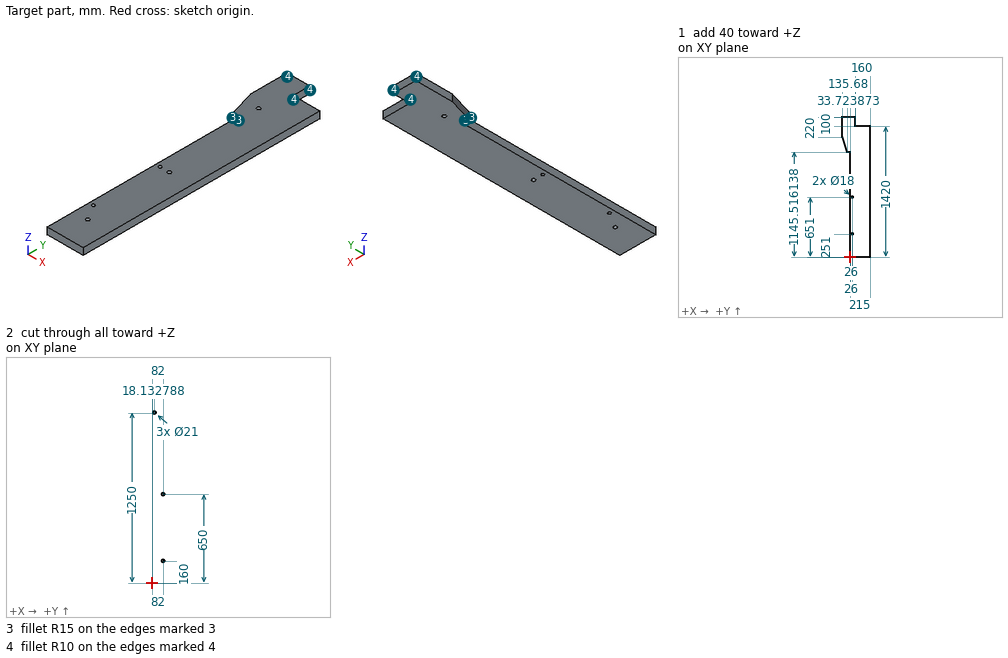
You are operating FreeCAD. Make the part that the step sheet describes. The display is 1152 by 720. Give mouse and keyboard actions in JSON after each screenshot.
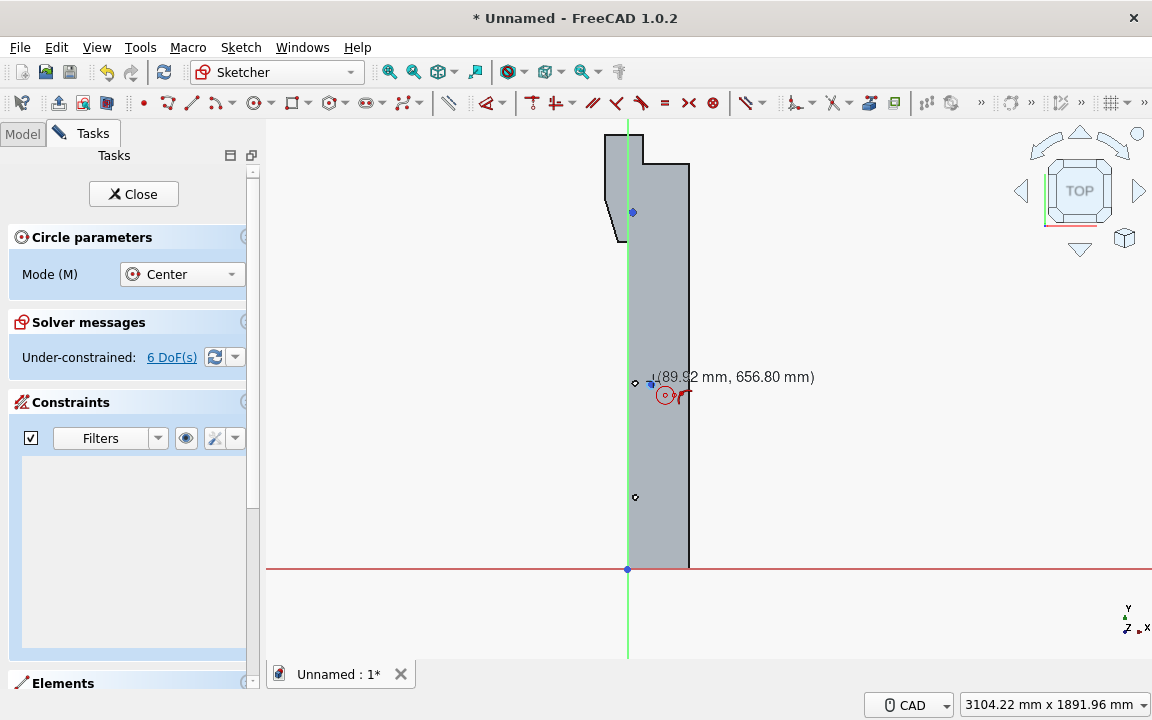
{"action": "scroll", "coordinate": [651, 523], "scroll_direction": "up", "scroll_amount": 11}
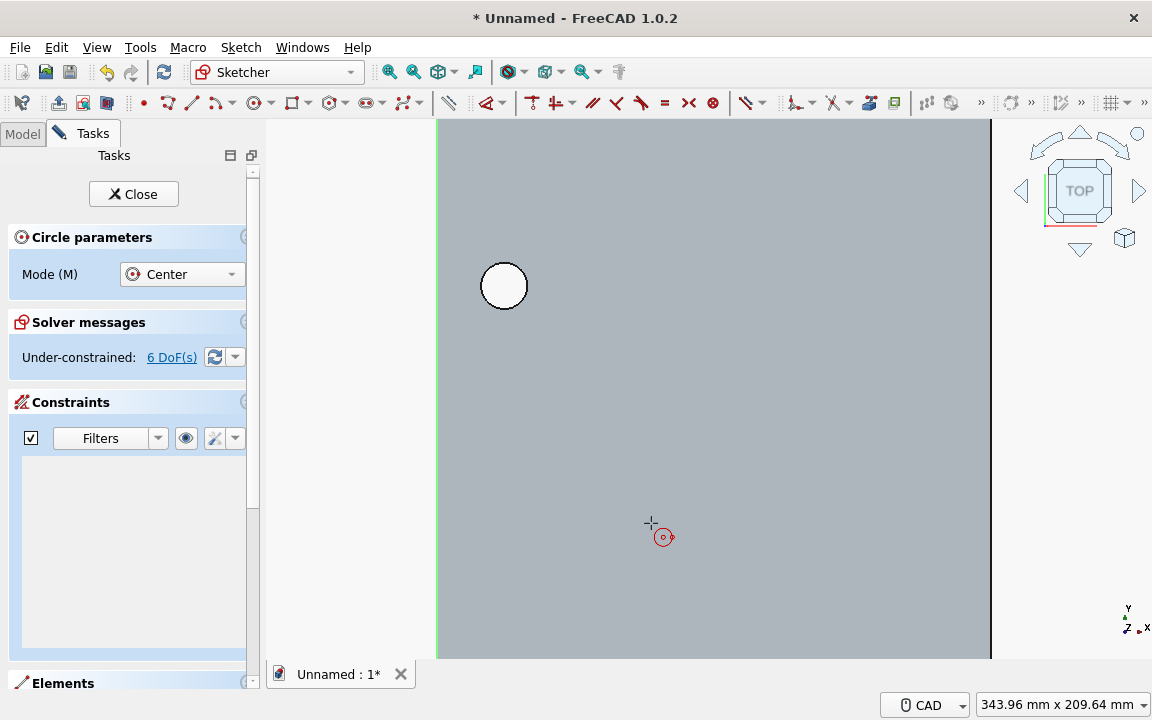
{"action": "scroll", "coordinate": [651, 524], "scroll_direction": "down", "scroll_amount": 11}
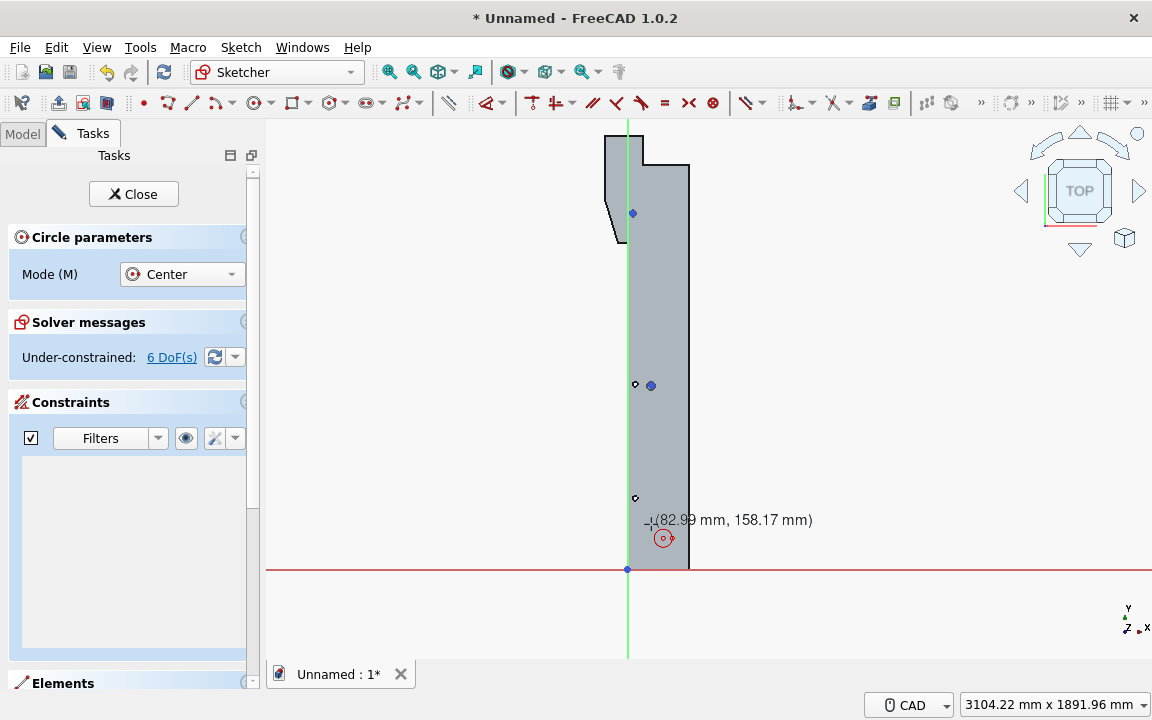
{"action": "left_click", "coordinate": [651, 524]}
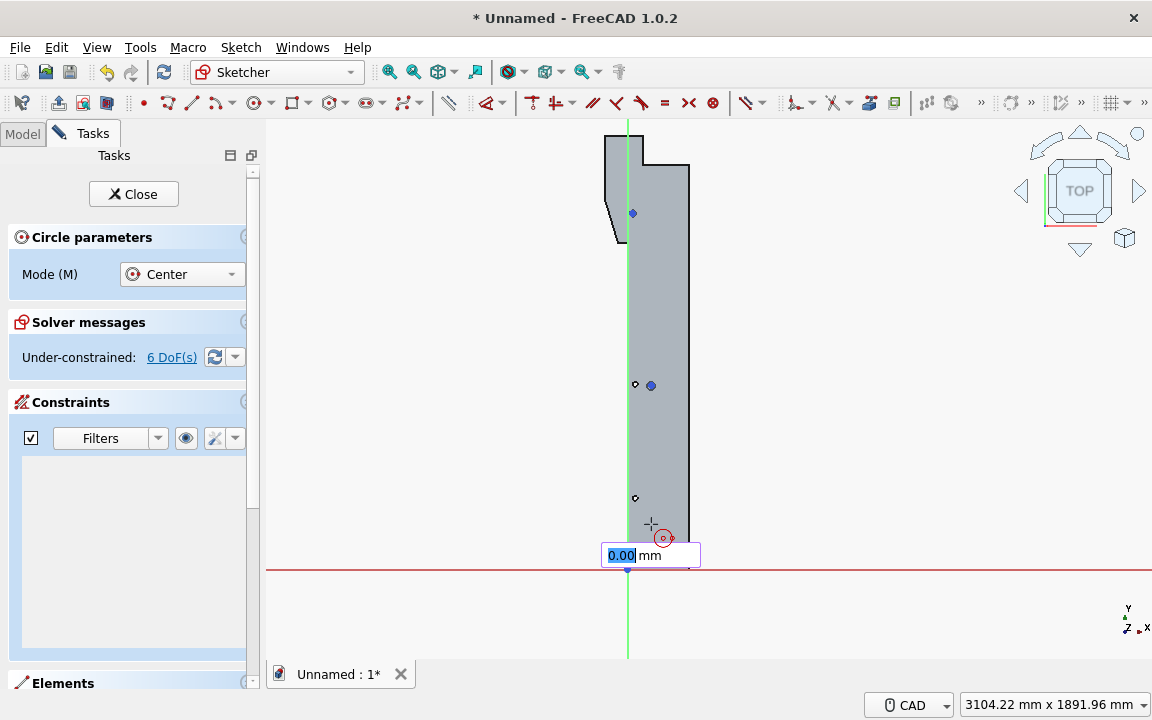
{"action": "scroll", "coordinate": [653, 522], "scroll_direction": "up", "scroll_amount": 9}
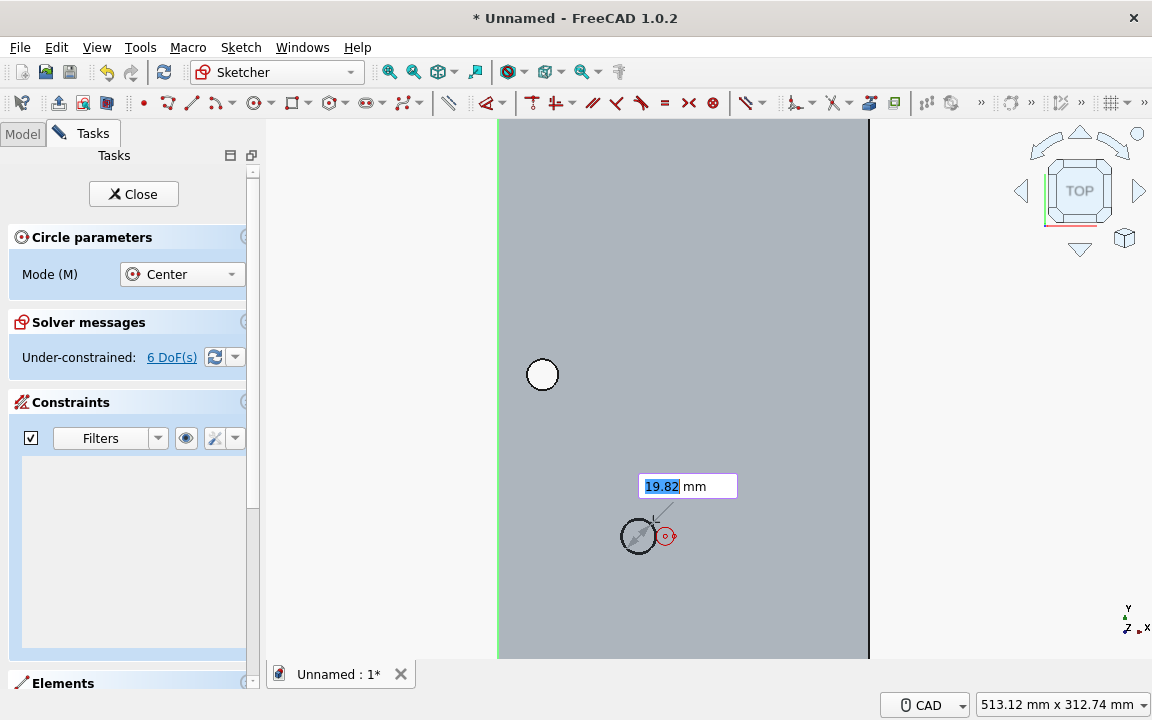
{"action": "left_click", "coordinate": [652, 519]}
{"action": "key", "text": "Escape"}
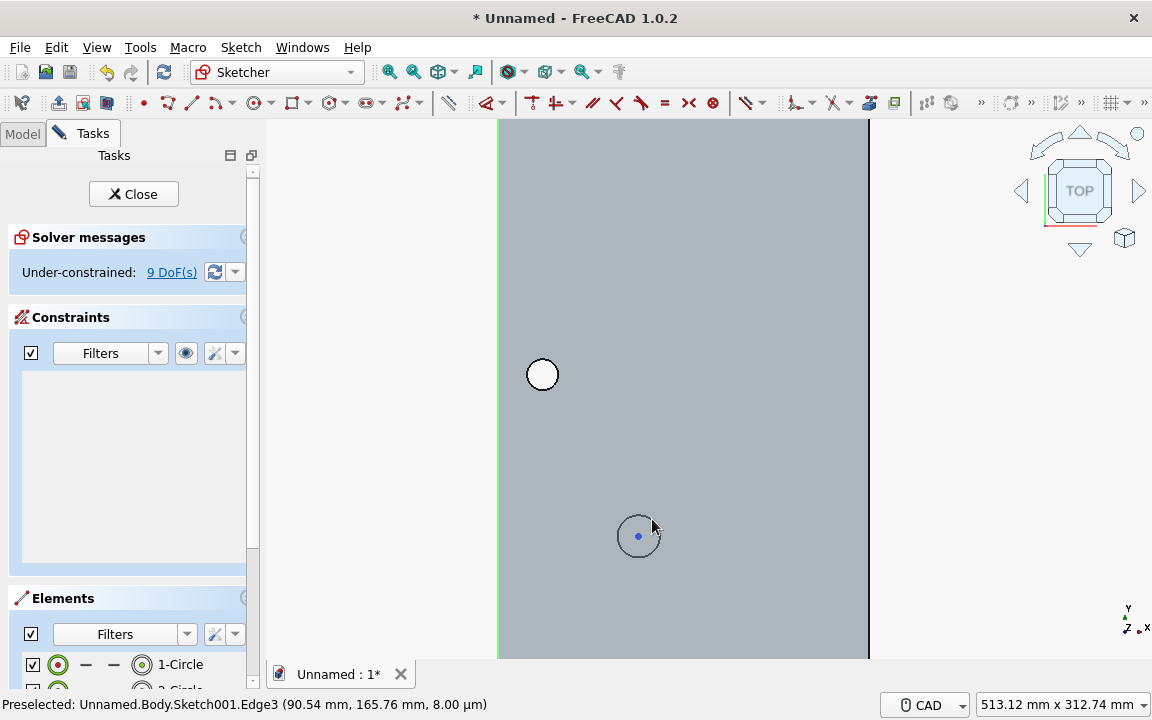
{"action": "scroll", "coordinate": [653, 522], "scroll_direction": "down", "scroll_amount": 9}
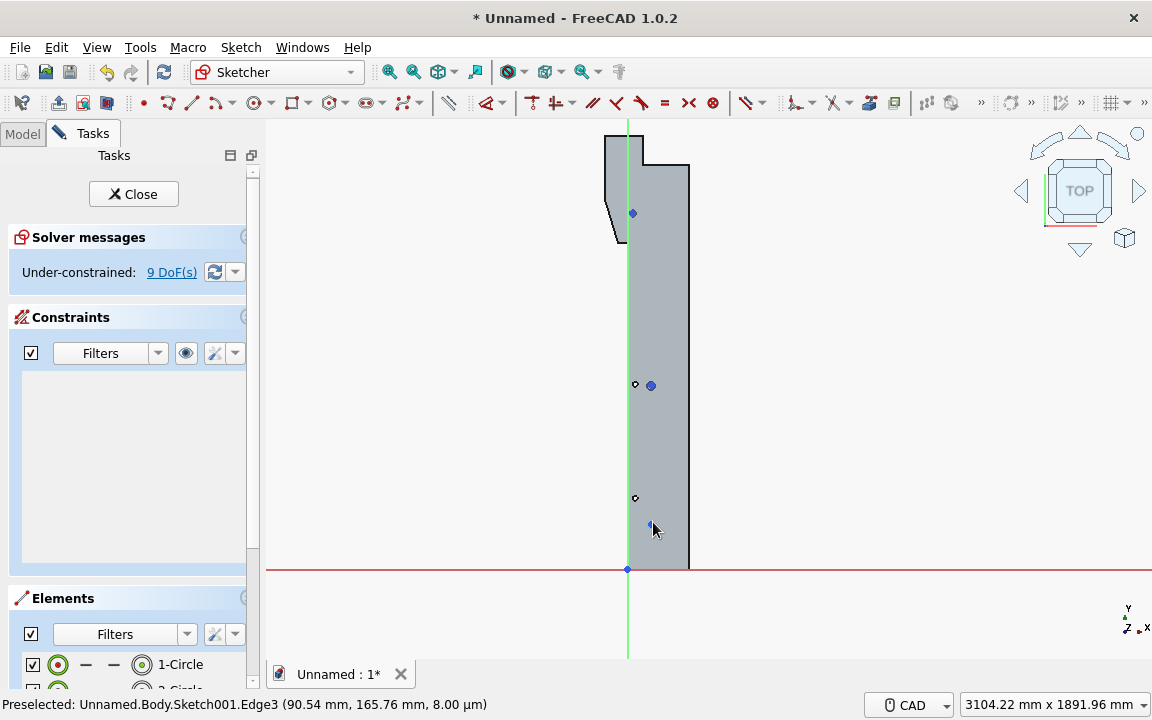
{"action": "scroll", "coordinate": [635, 211], "scroll_direction": "up", "scroll_amount": 8}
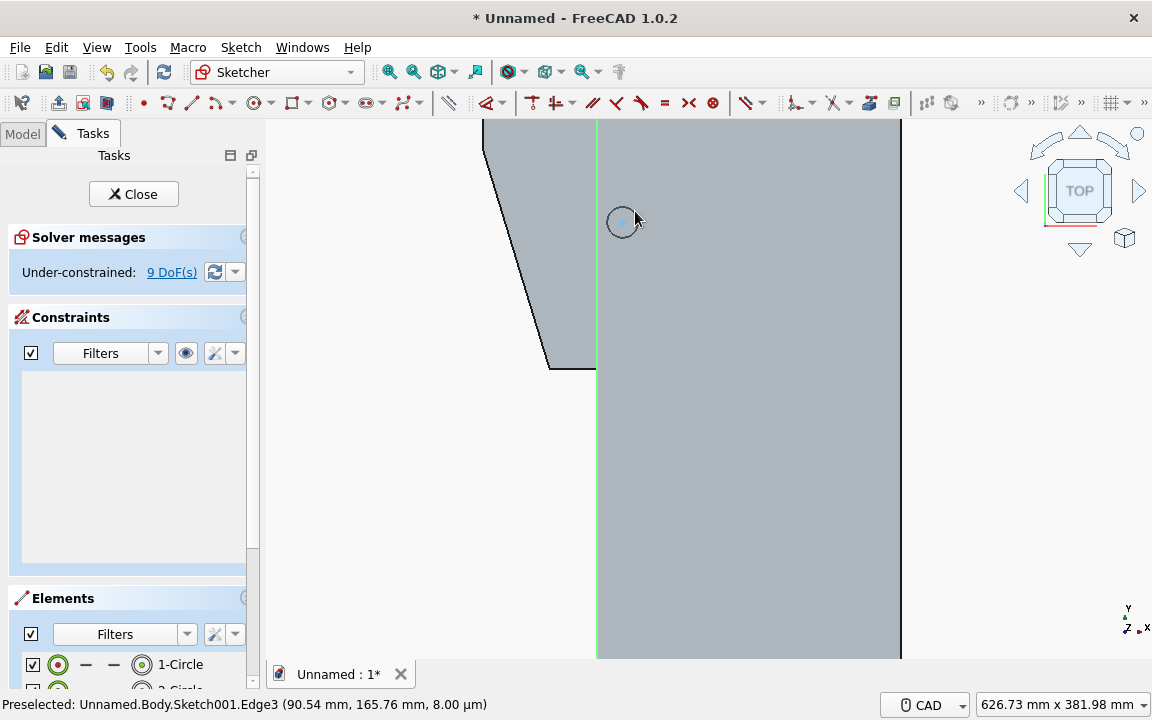
{"action": "left_click", "coordinate": [634, 211]}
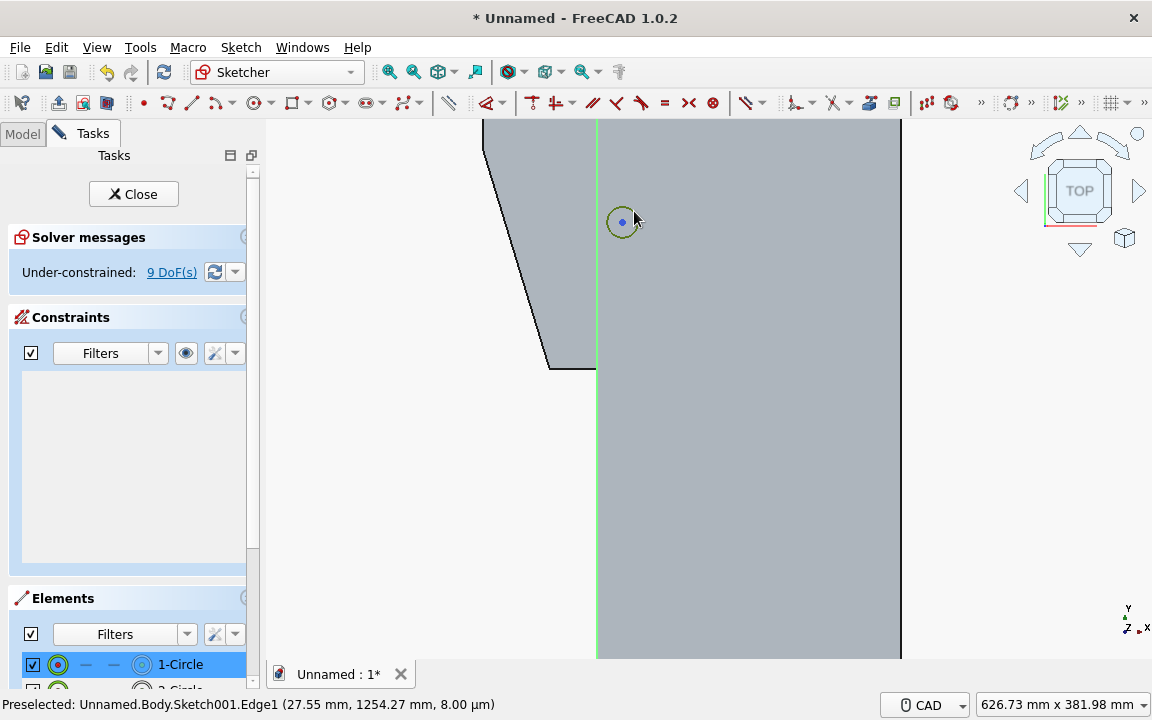
{"action": "scroll", "coordinate": [635, 210], "scroll_direction": "down", "scroll_amount": 8}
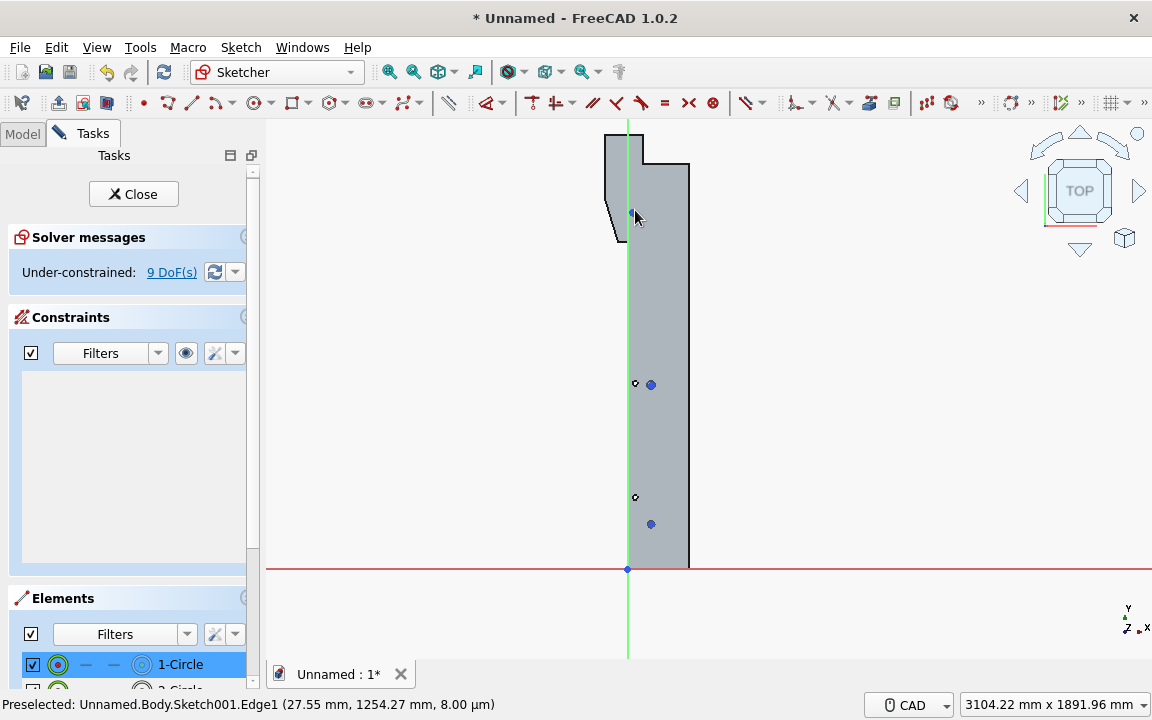
{"action": "scroll", "coordinate": [654, 382], "scroll_direction": "up", "scroll_amount": 7}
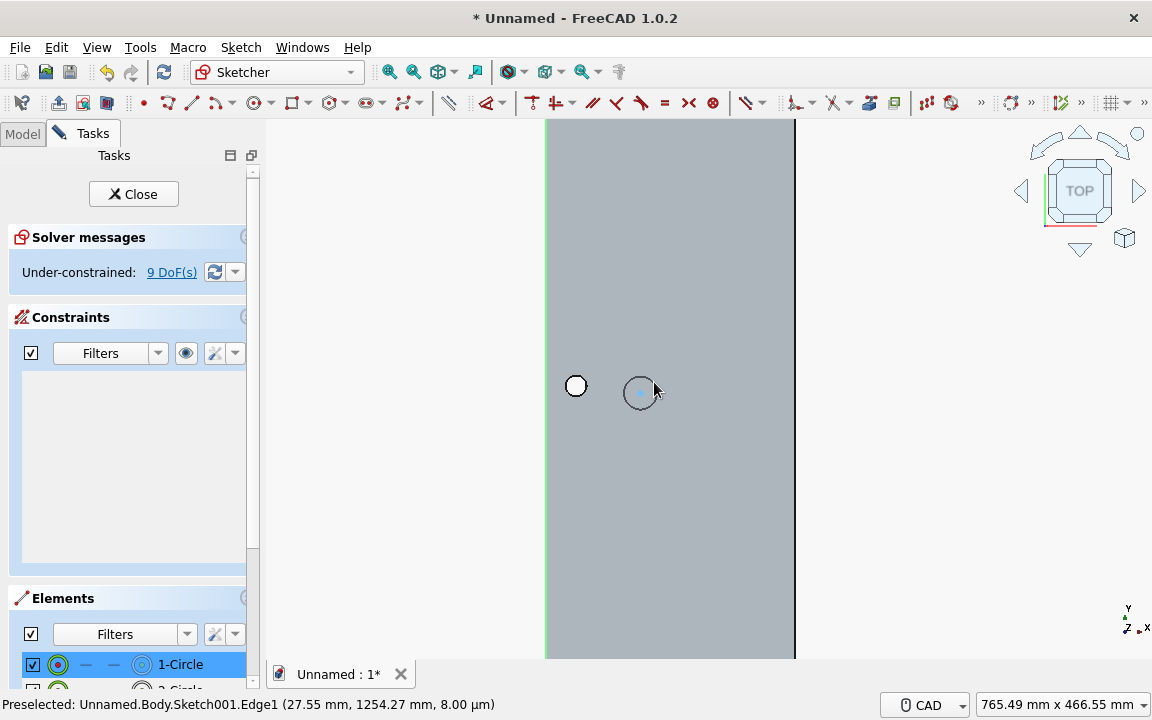
{"action": "left_click", "coordinate": [652, 381]}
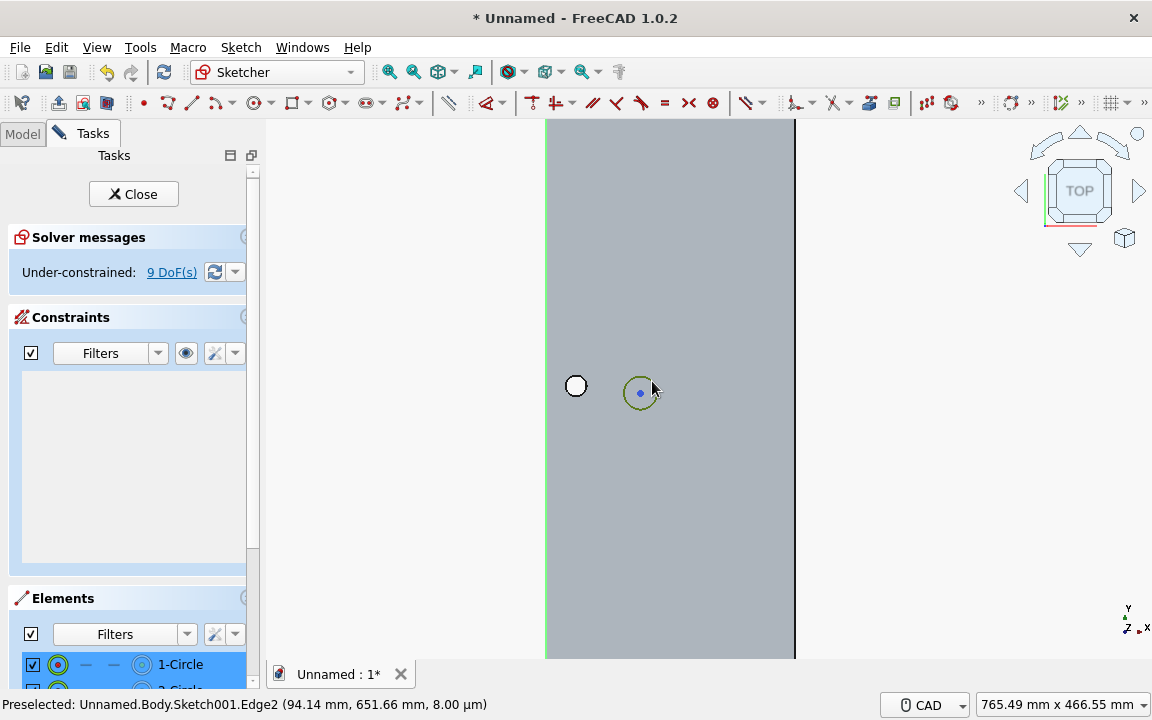
{"action": "scroll", "coordinate": [654, 382], "scroll_direction": "down", "scroll_amount": 7}